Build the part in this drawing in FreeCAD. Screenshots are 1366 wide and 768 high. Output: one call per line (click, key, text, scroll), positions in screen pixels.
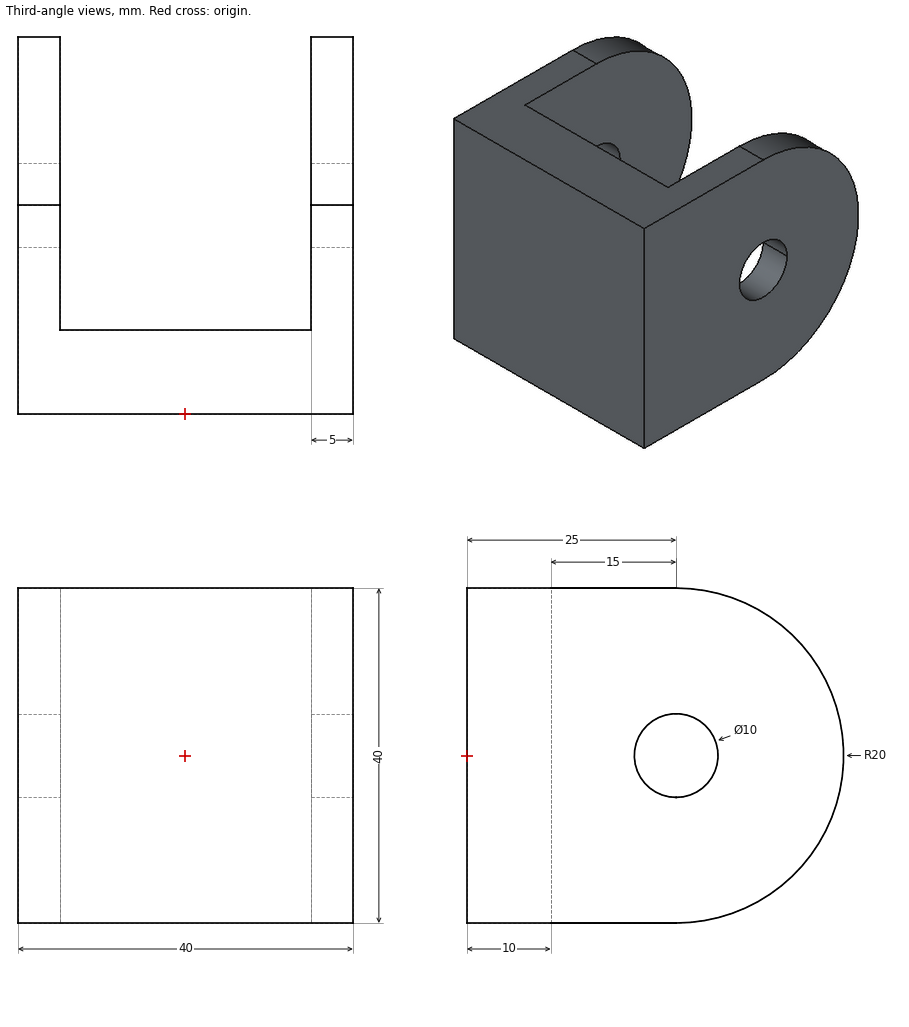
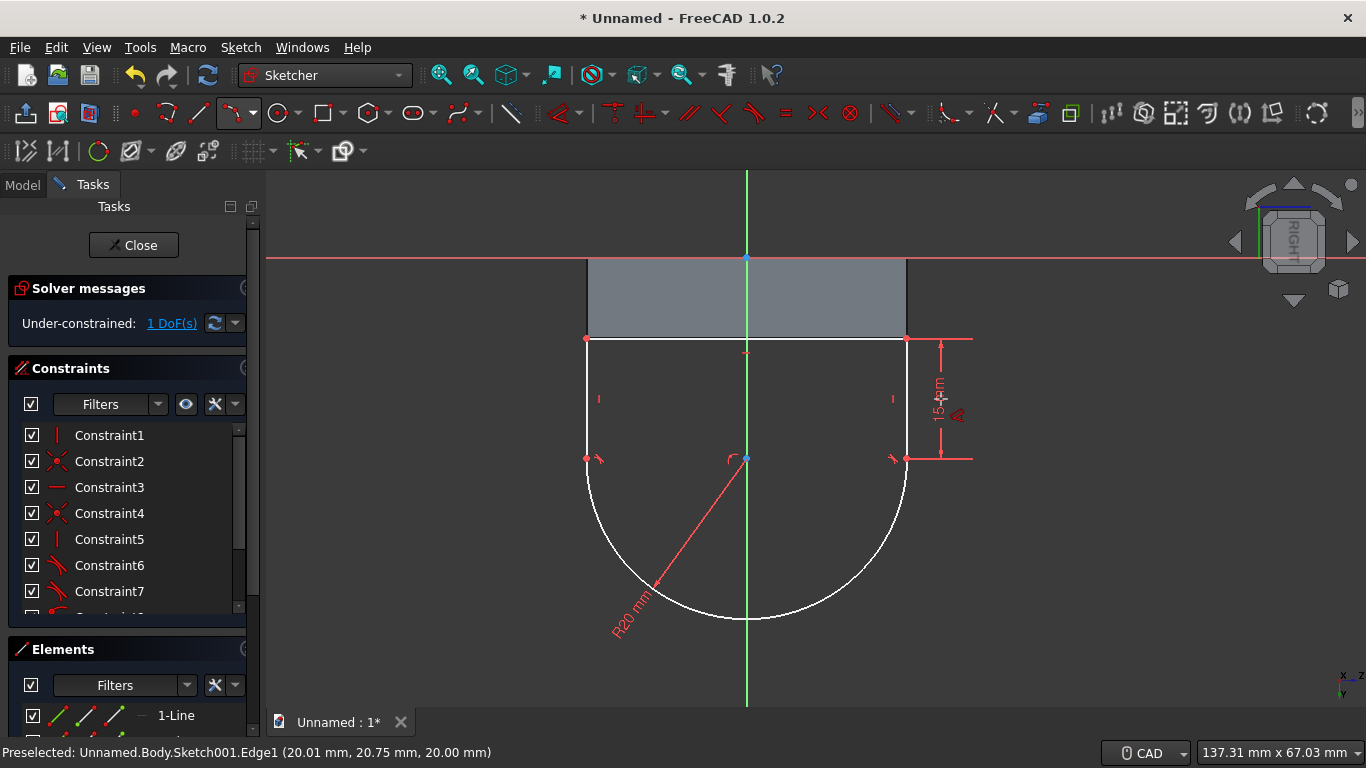
click(907, 459)
click(941, 358)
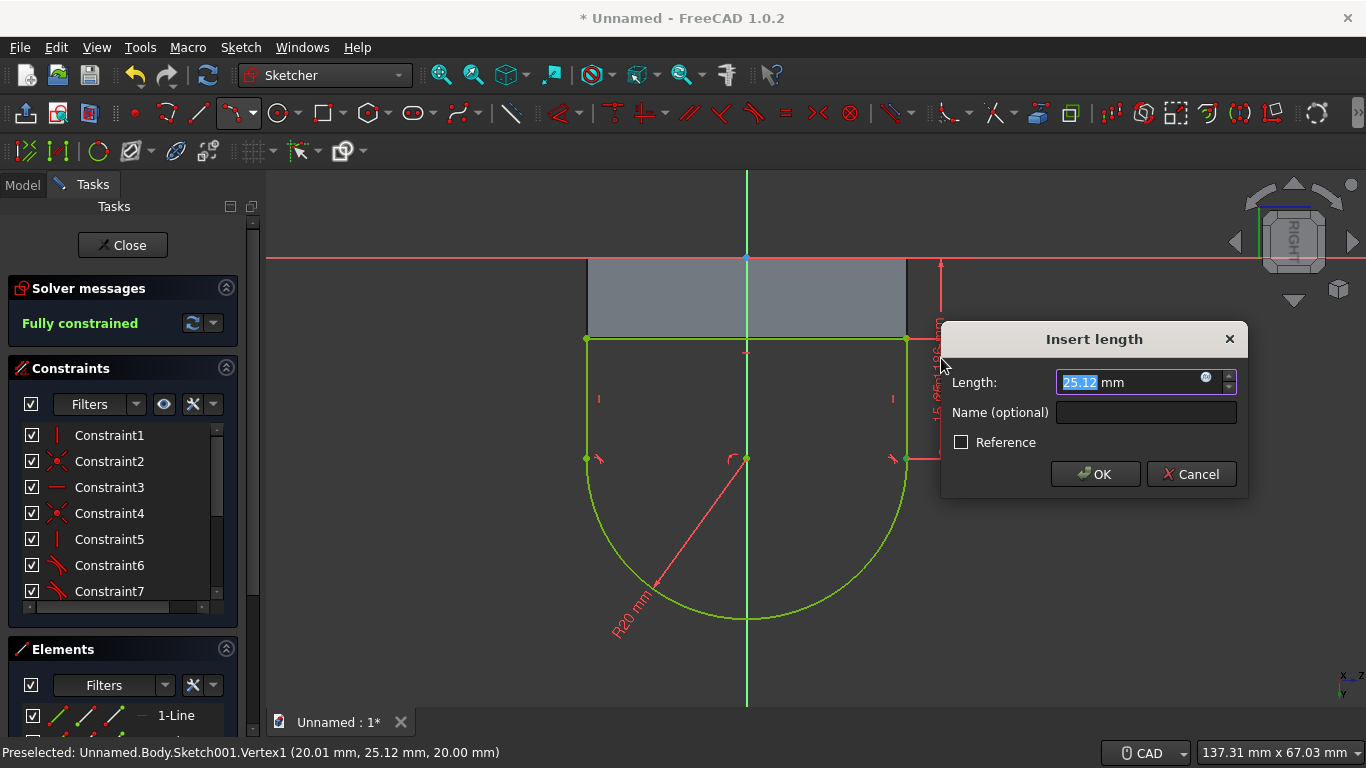
text(25)
key(Return)
key(Escape)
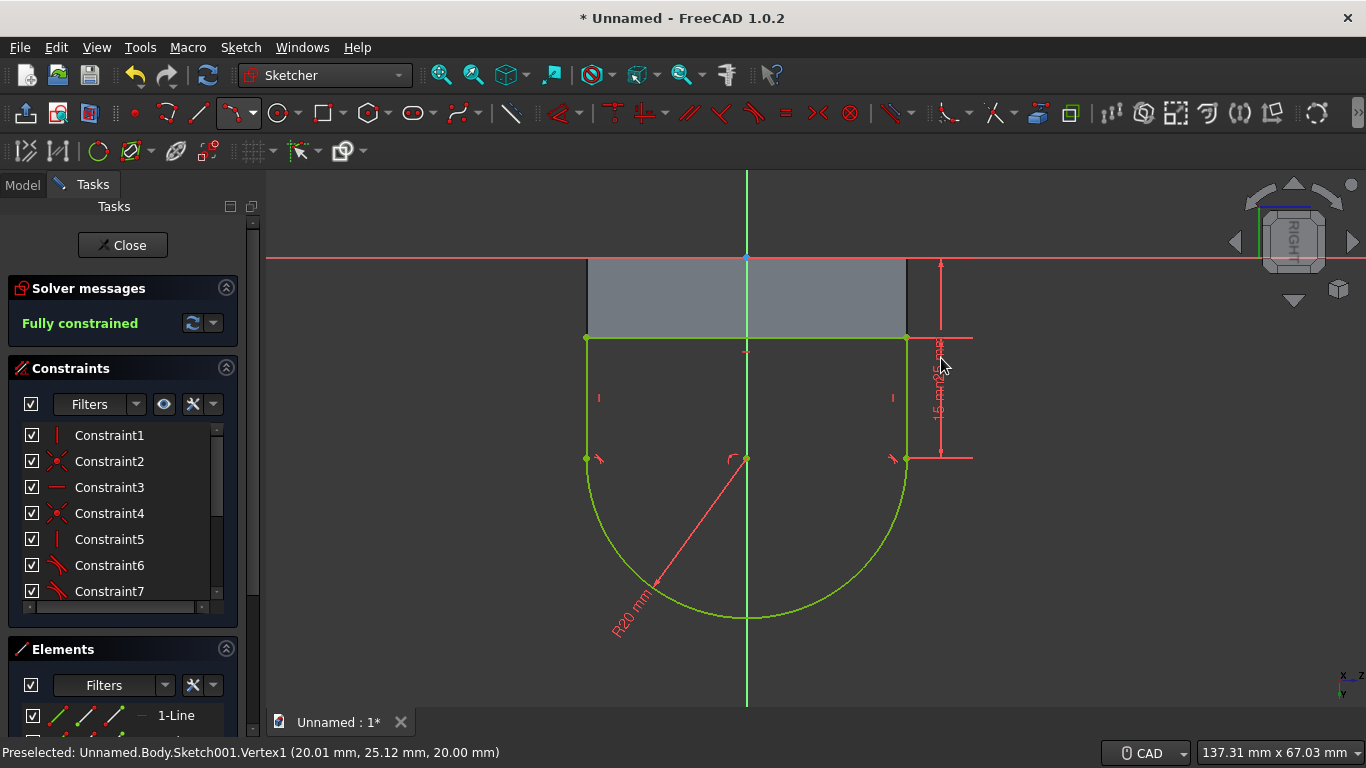
click(123, 245)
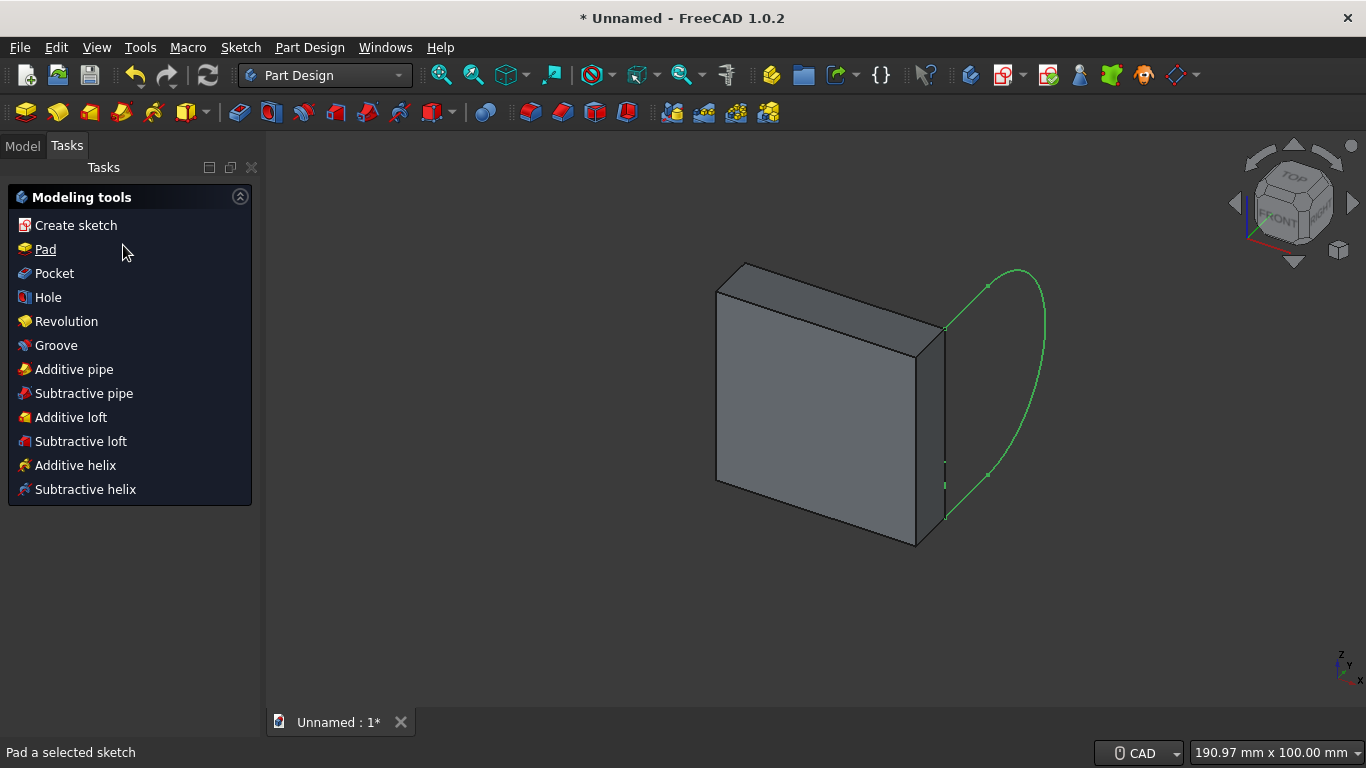
click(26, 112)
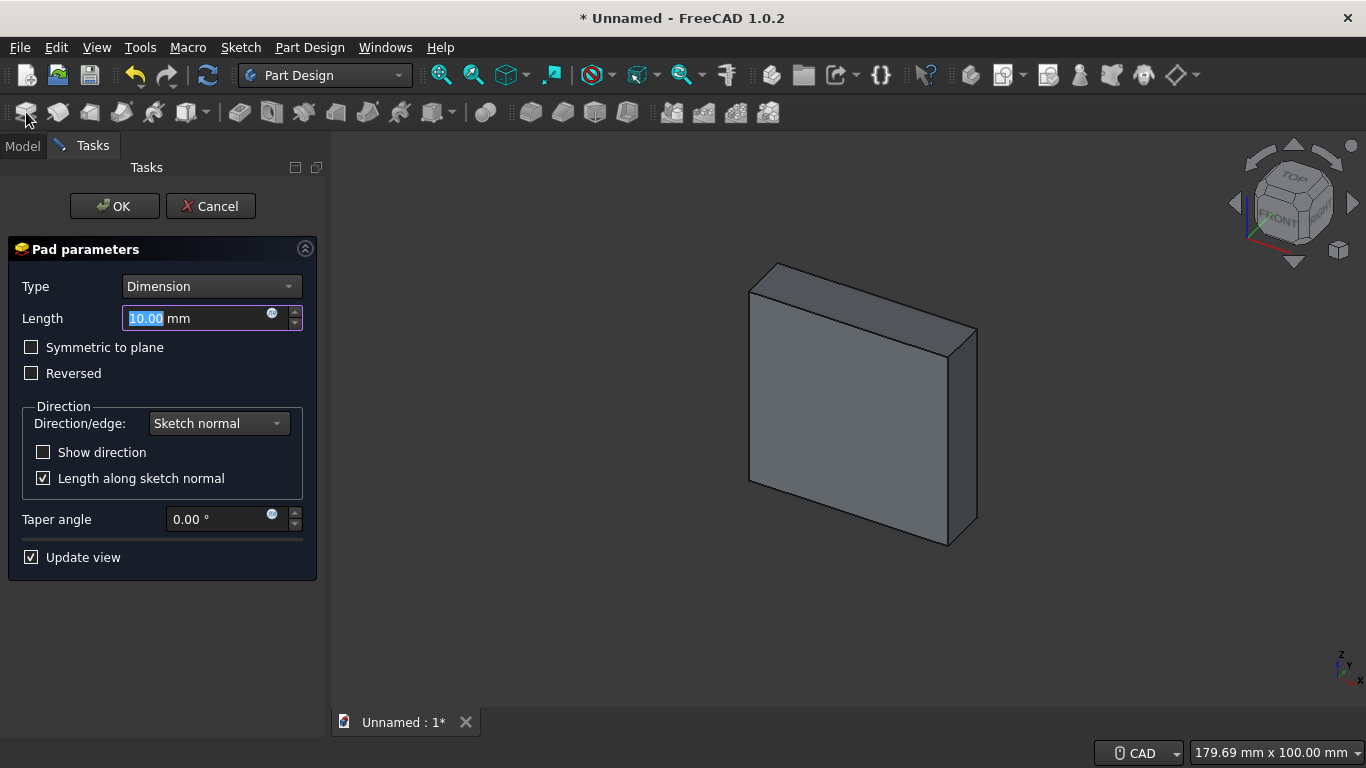
text(5)
key(Tab)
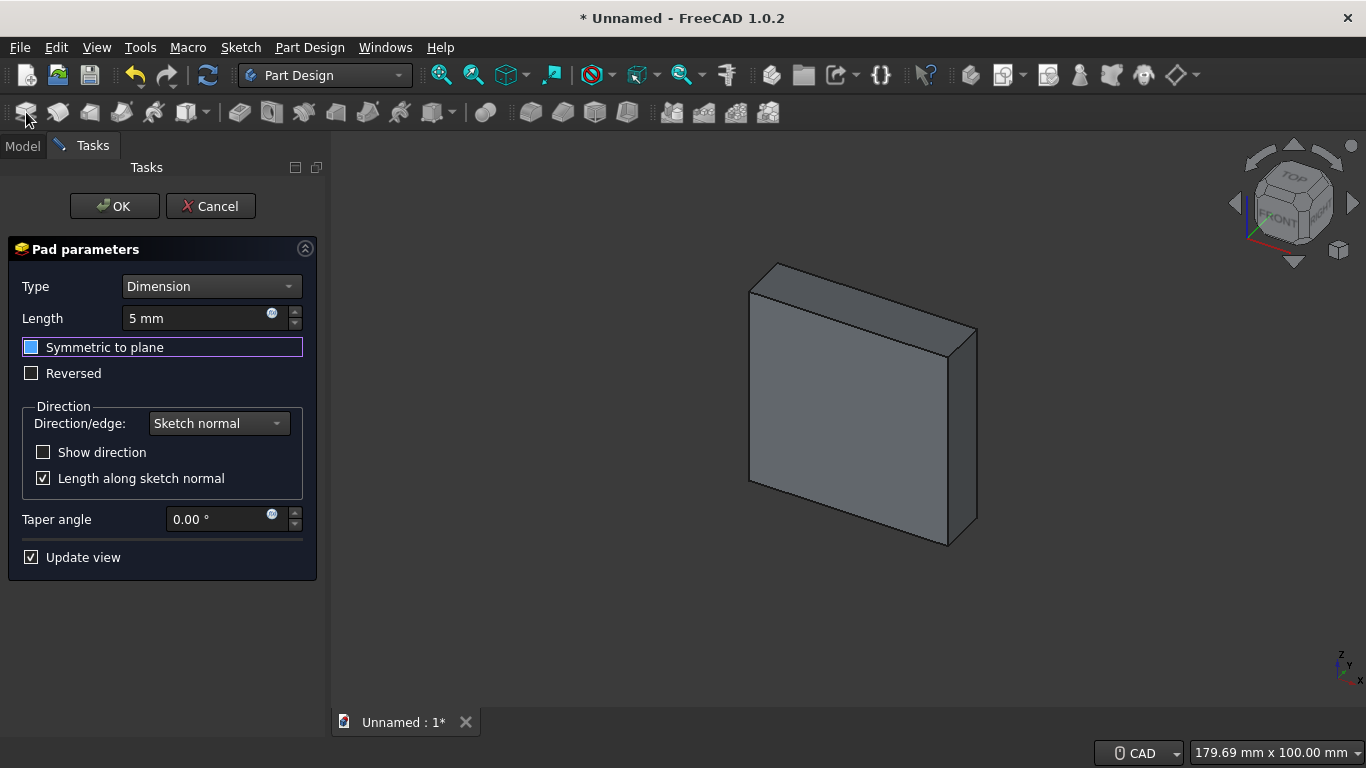
click(30, 373)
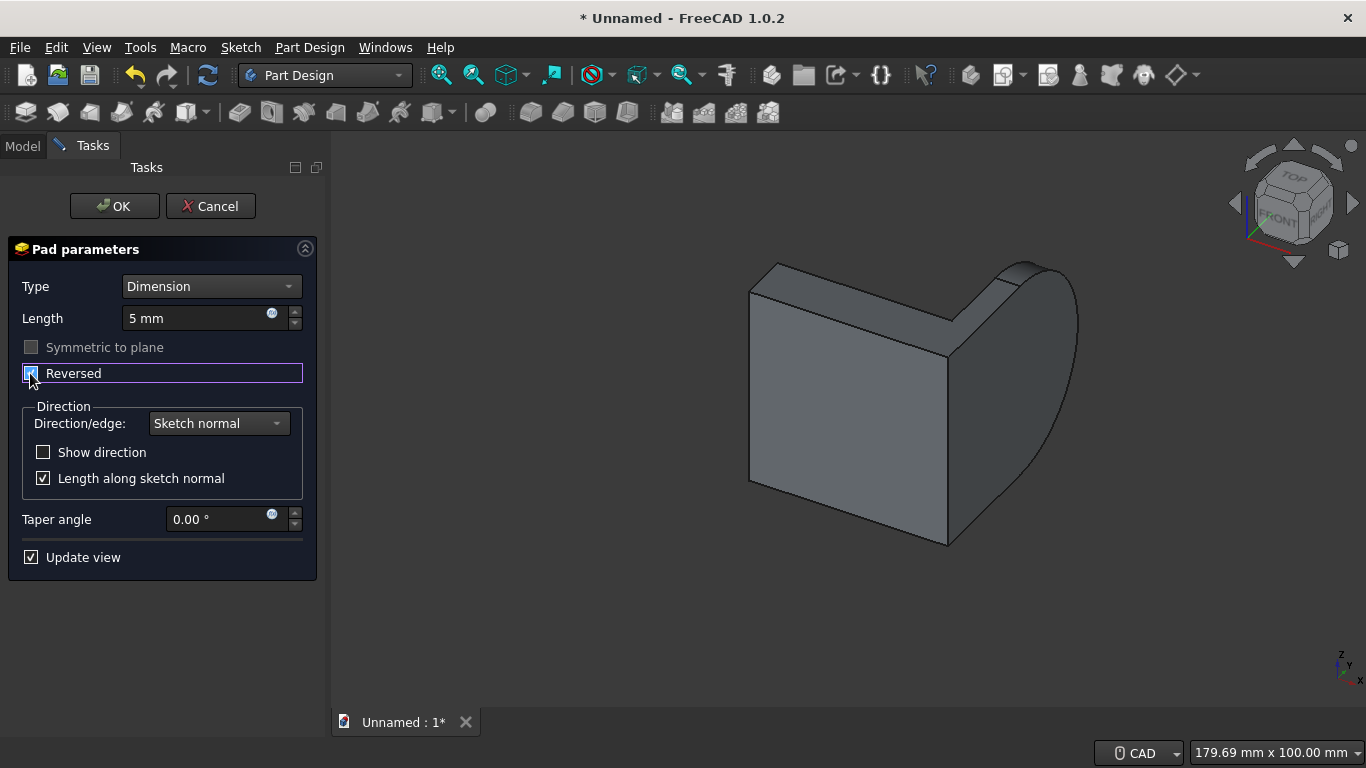
click(115, 206)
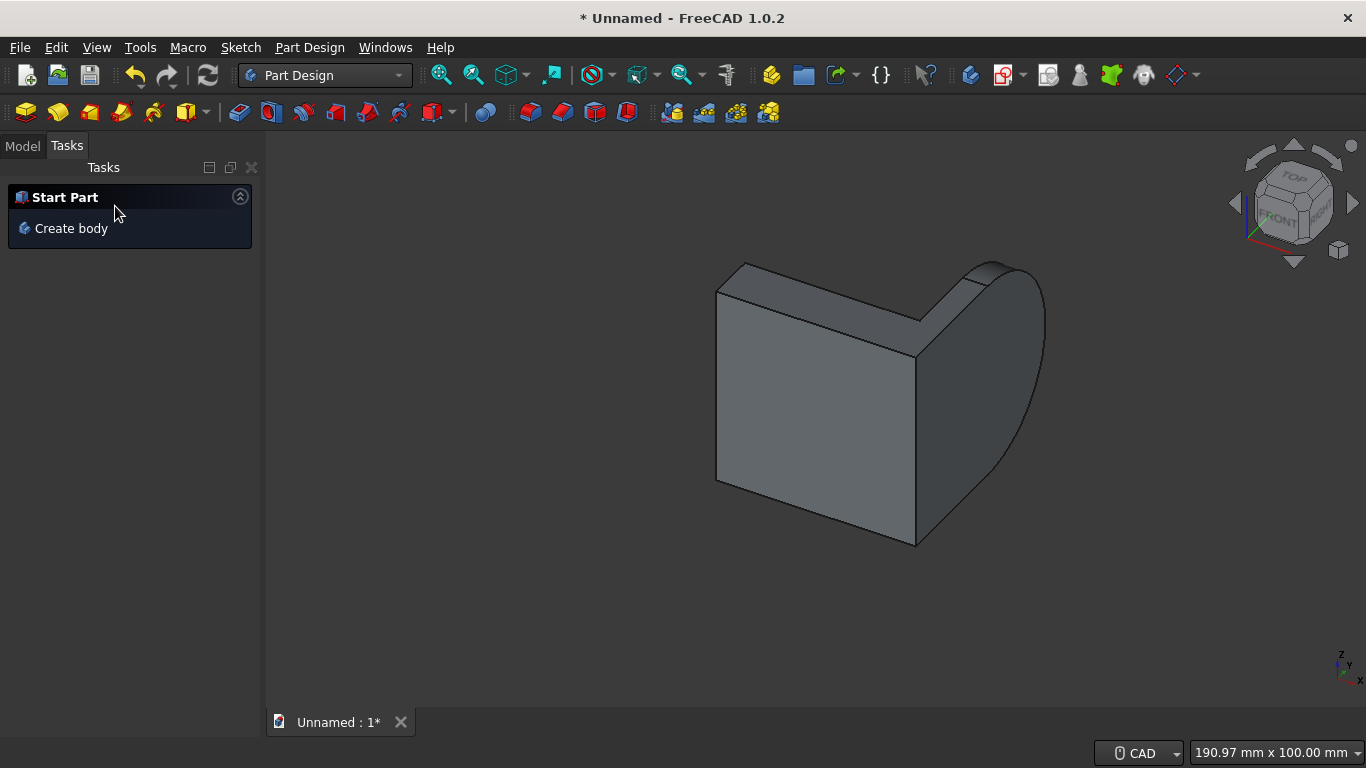
click(23, 145)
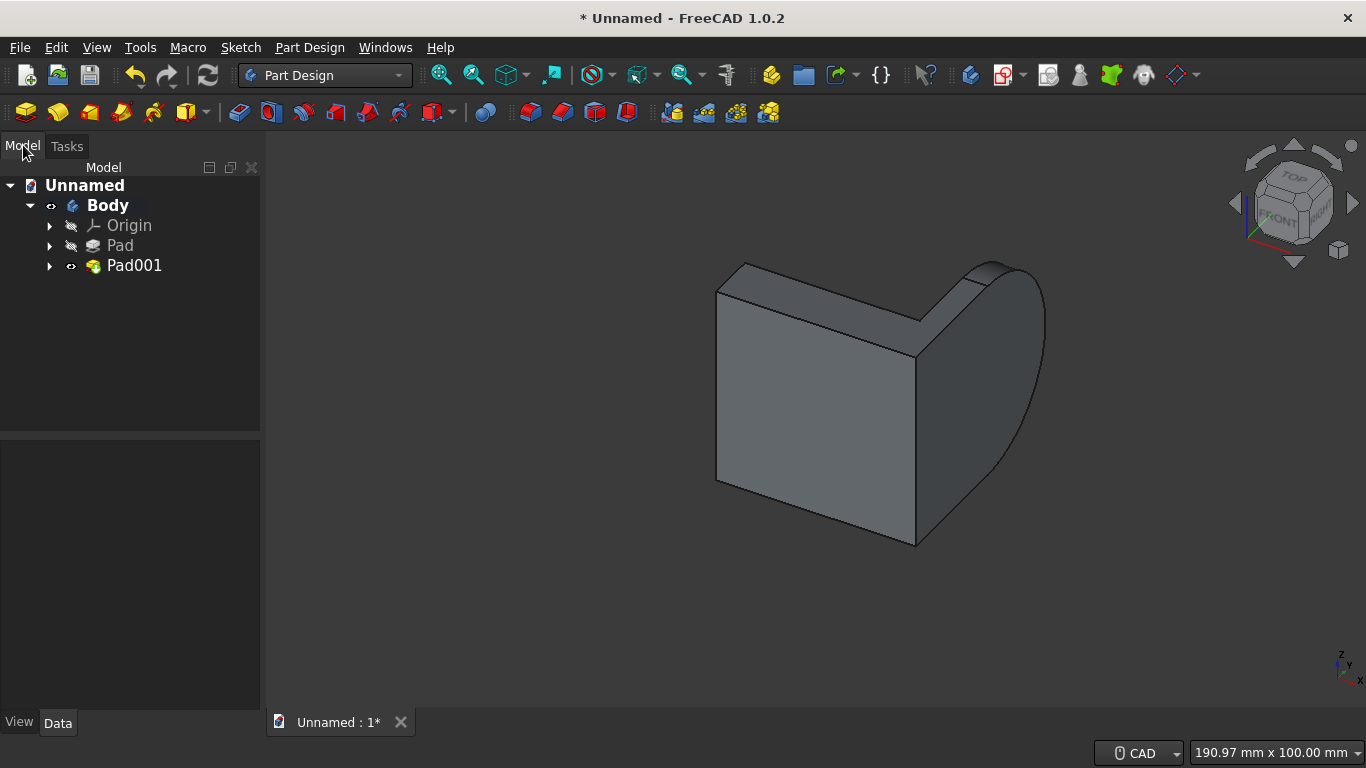
click(116, 266)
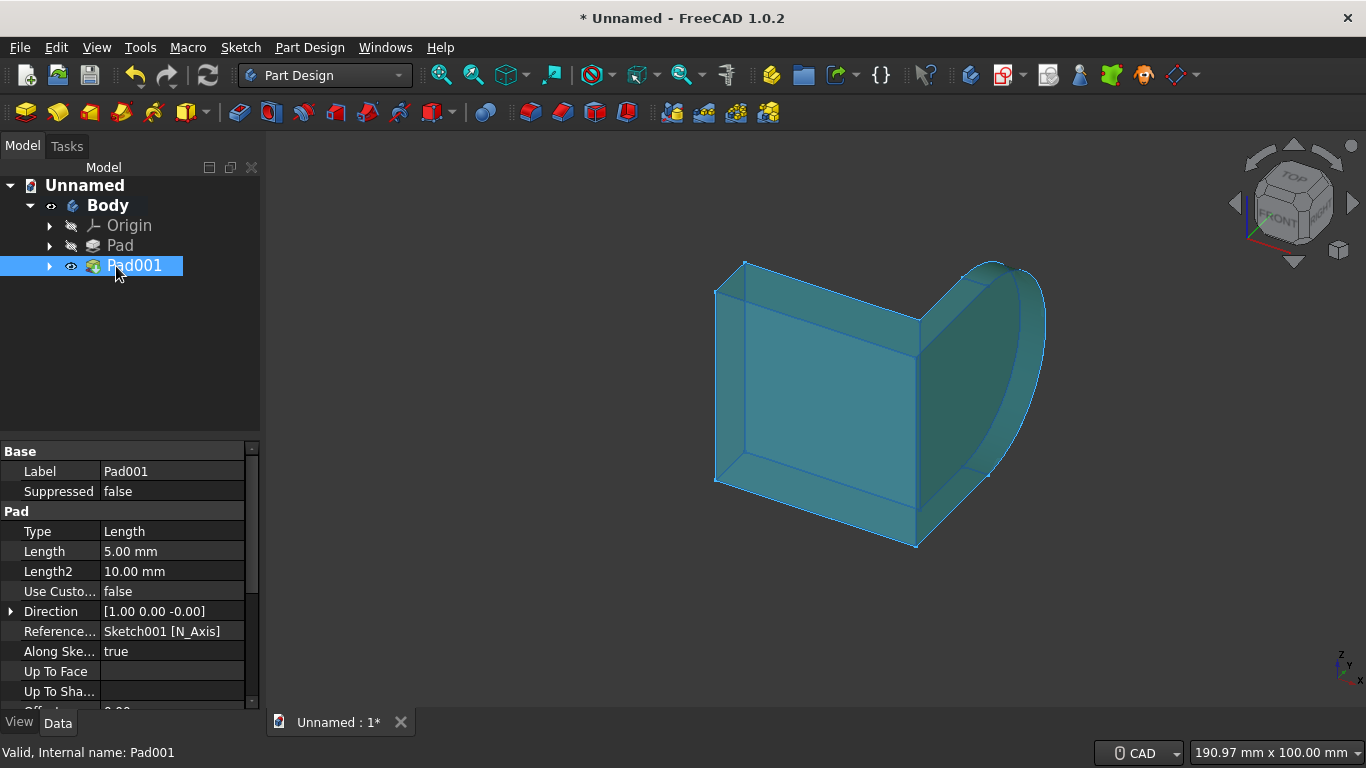
click(672, 112)